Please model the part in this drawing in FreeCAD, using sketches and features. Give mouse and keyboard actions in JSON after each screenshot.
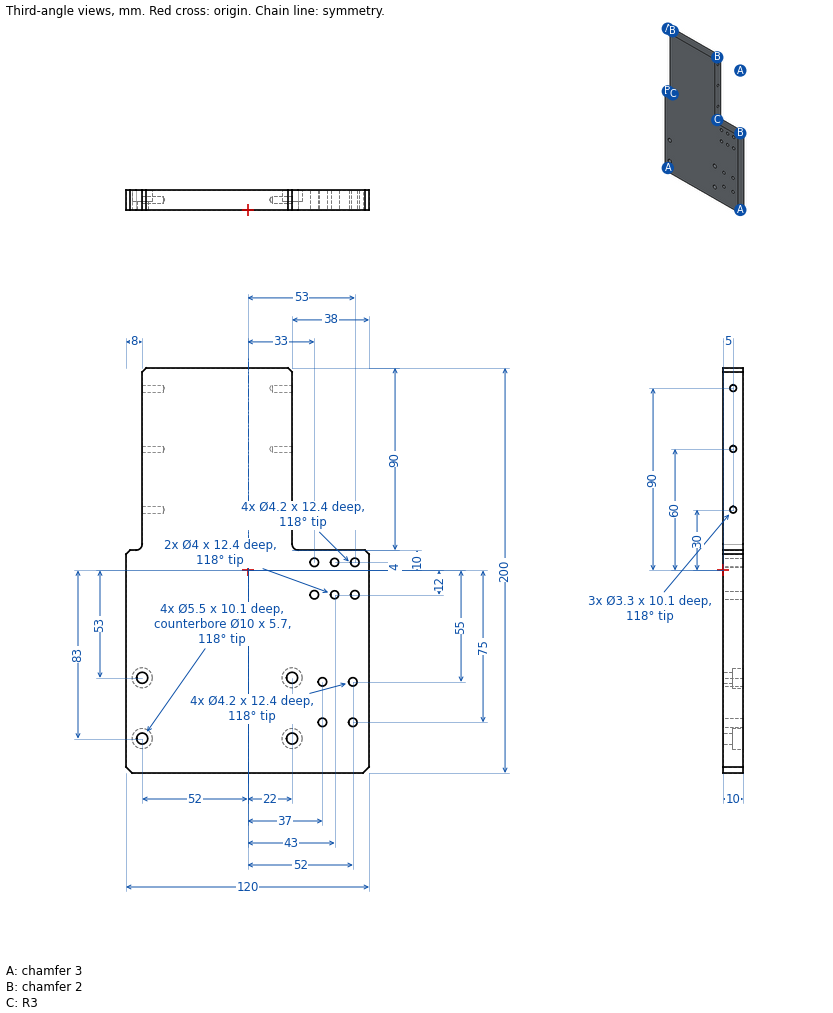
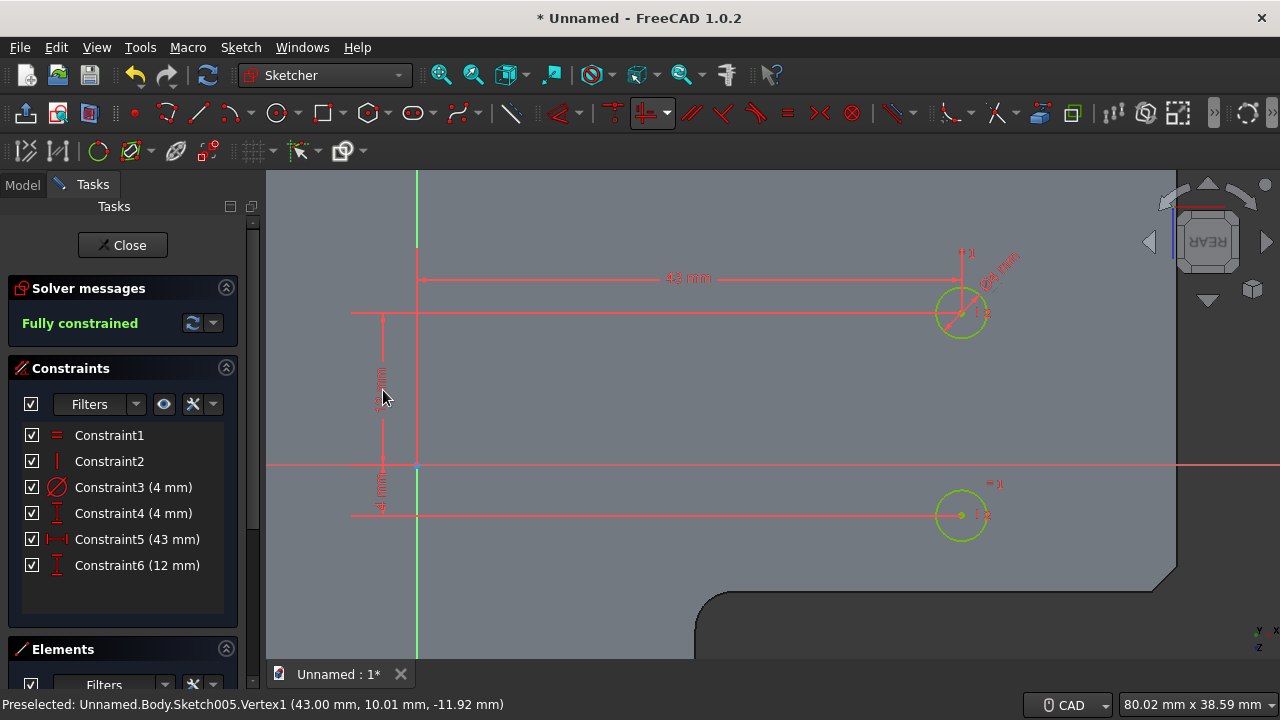
{"action": "left_click", "coordinate": [123, 245]}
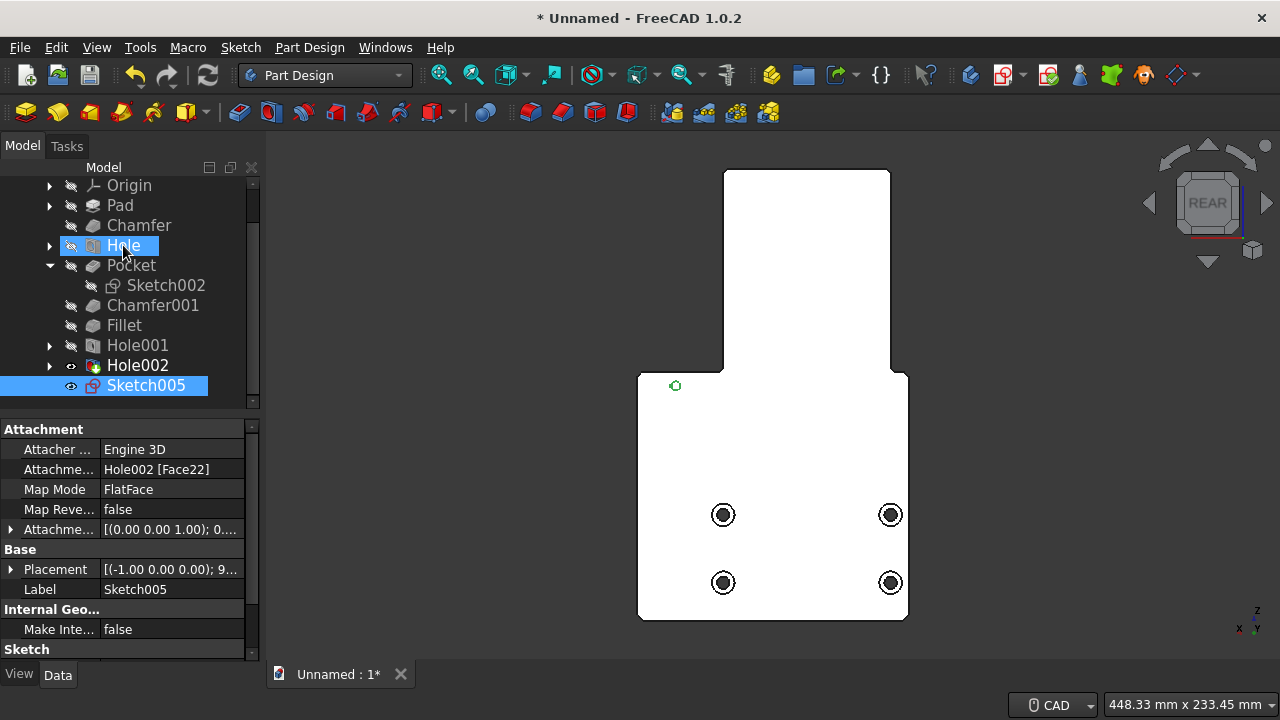
{"action": "left_click", "coordinate": [272, 112]}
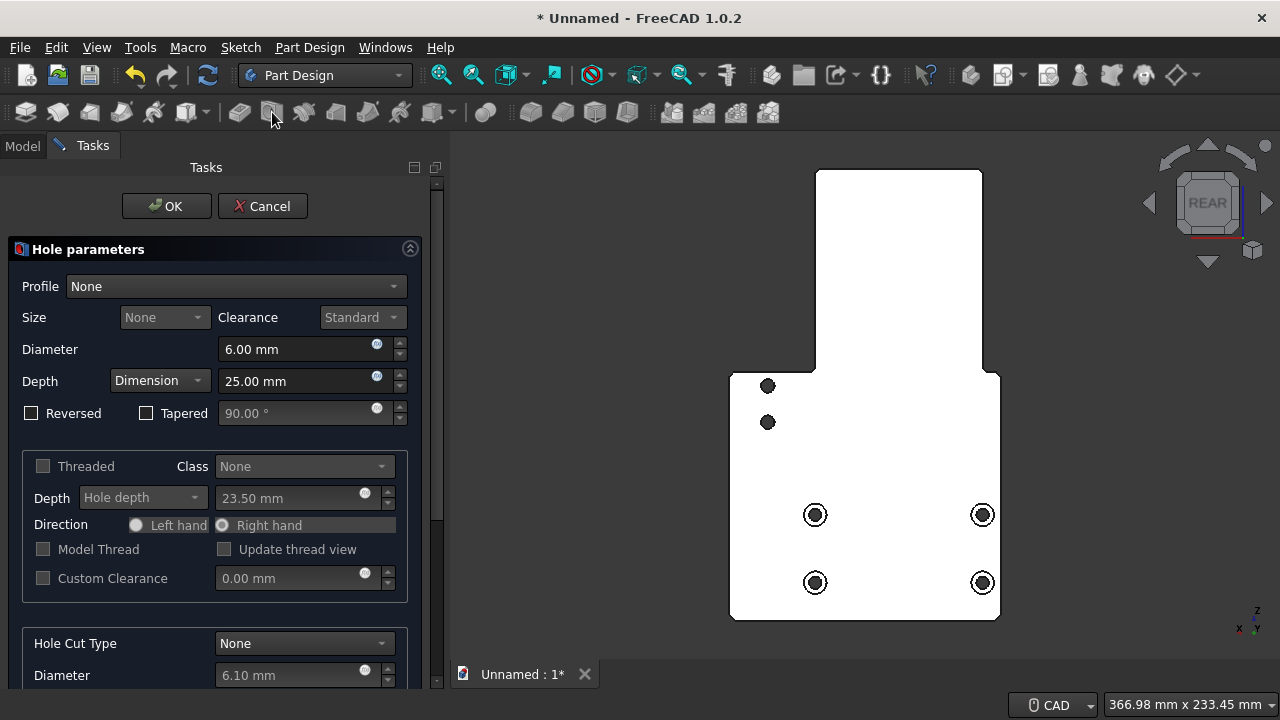
{"action": "triple_click", "coordinate": [305, 349]}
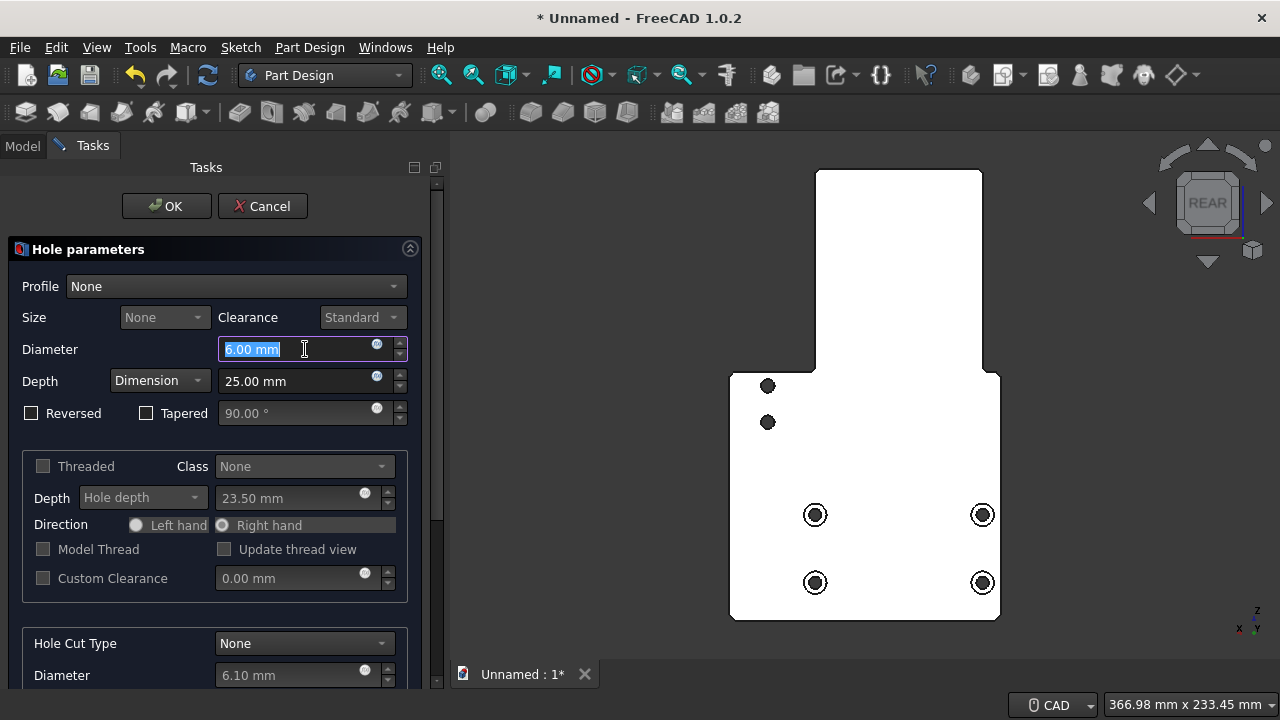
{"action": "type", "text": "4"}
{"action": "key", "text": "Tab"}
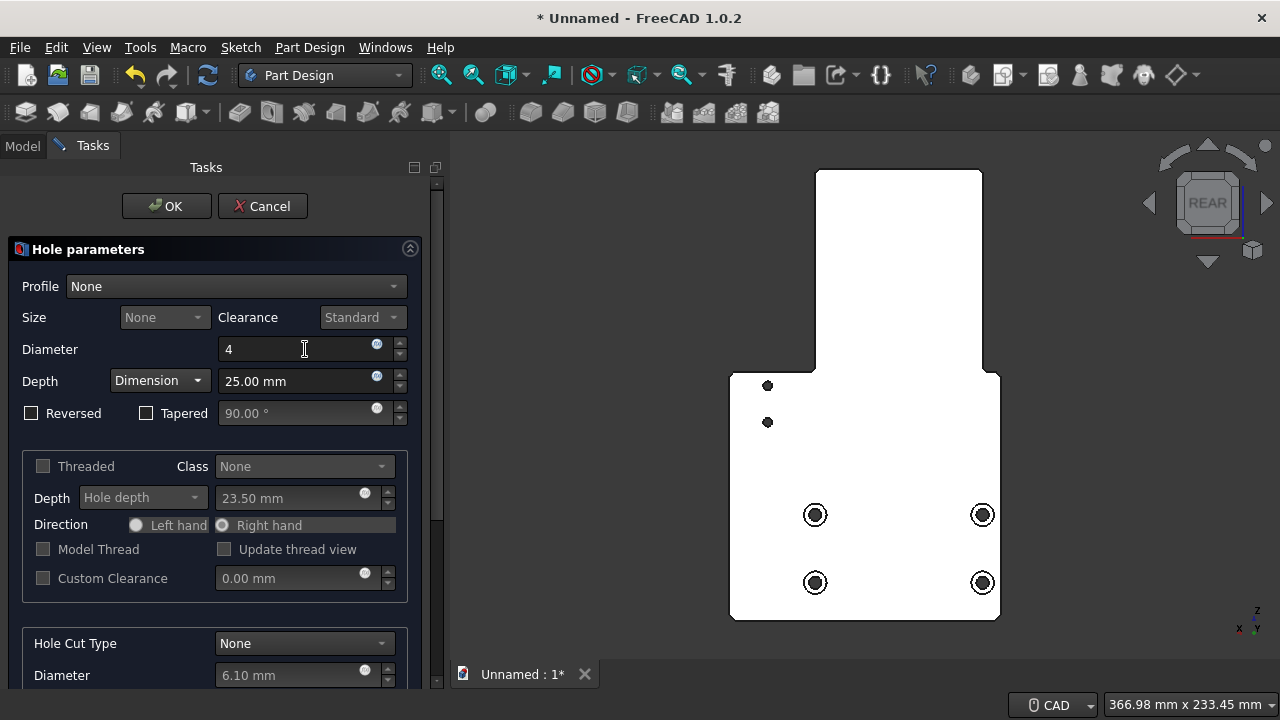
{"action": "triple_click", "coordinate": [305, 381]}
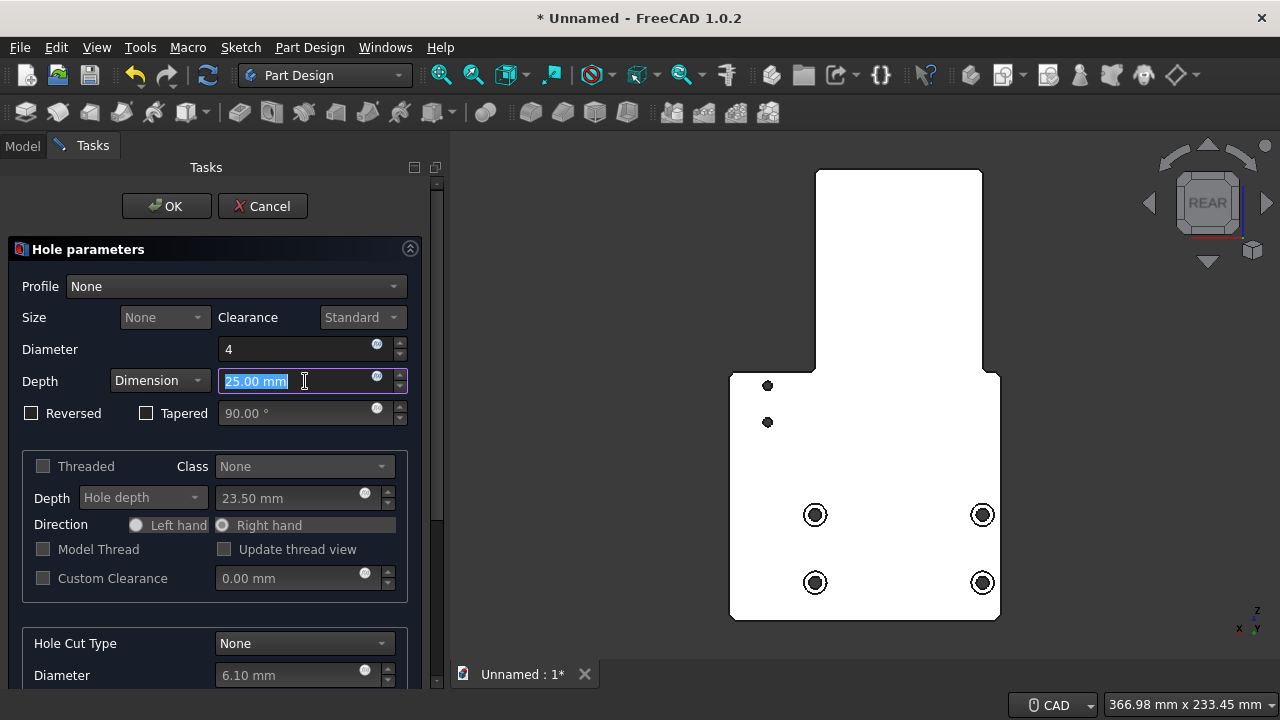
{"action": "type", "text": "12.4"}
{"action": "key", "text": "Tab"}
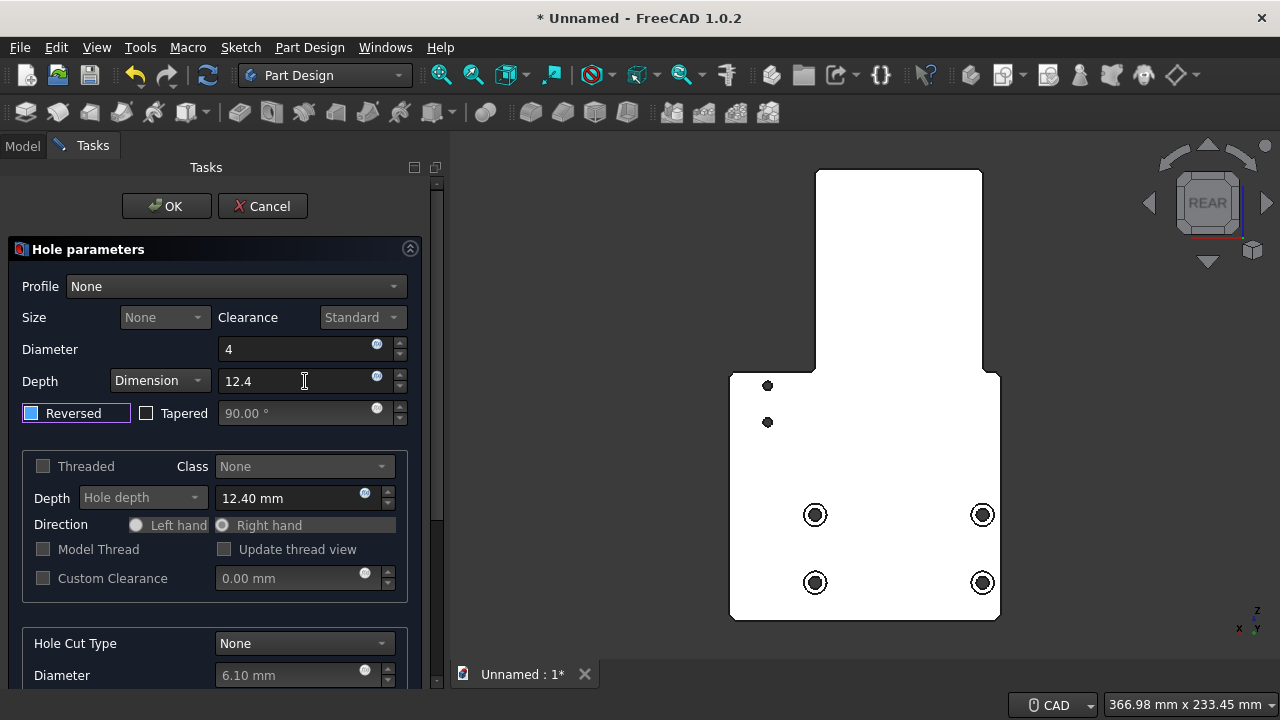
{"action": "left_click", "coordinate": [167, 206]}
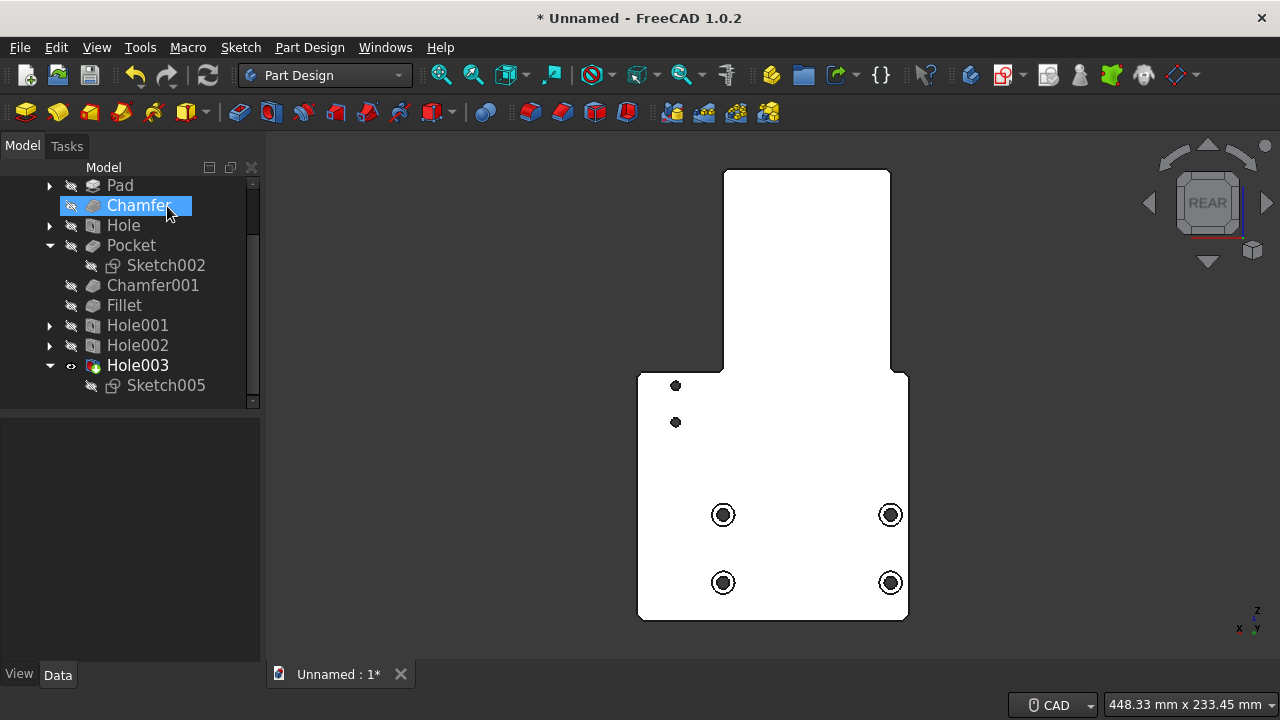
{"action": "left_click", "coordinate": [812, 459]}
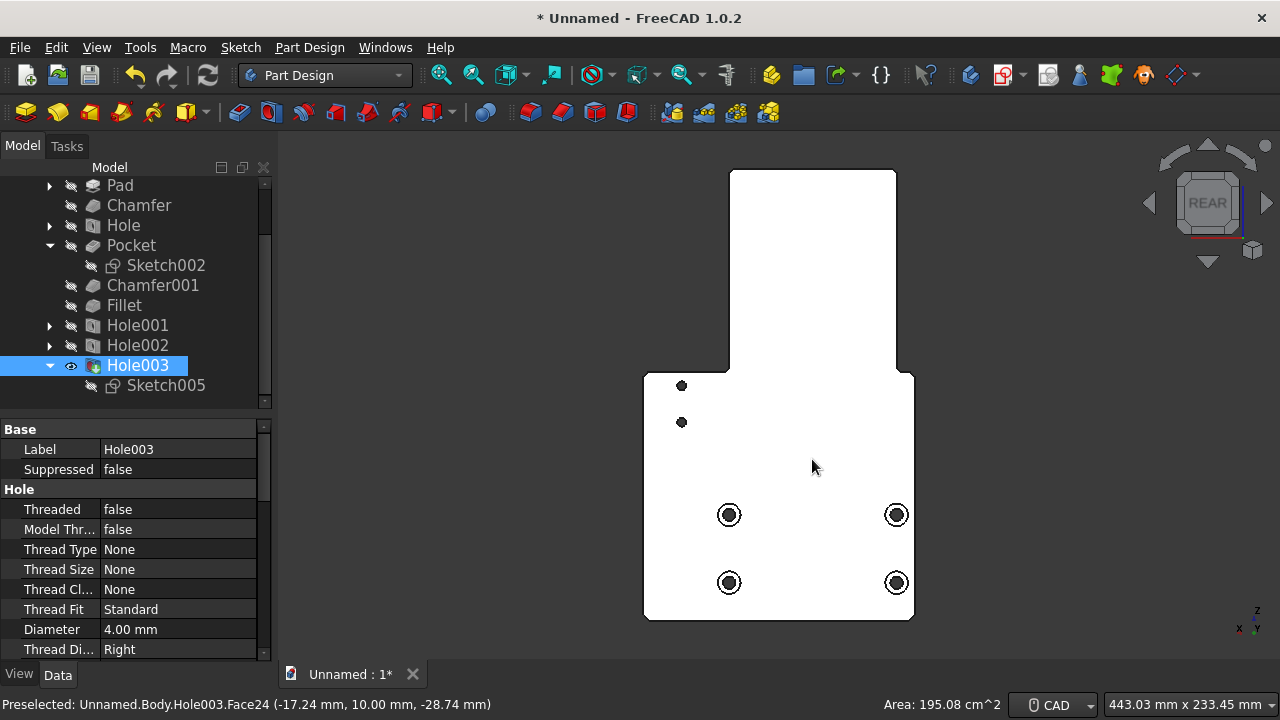
{"action": "left_click", "coordinate": [1004, 76]}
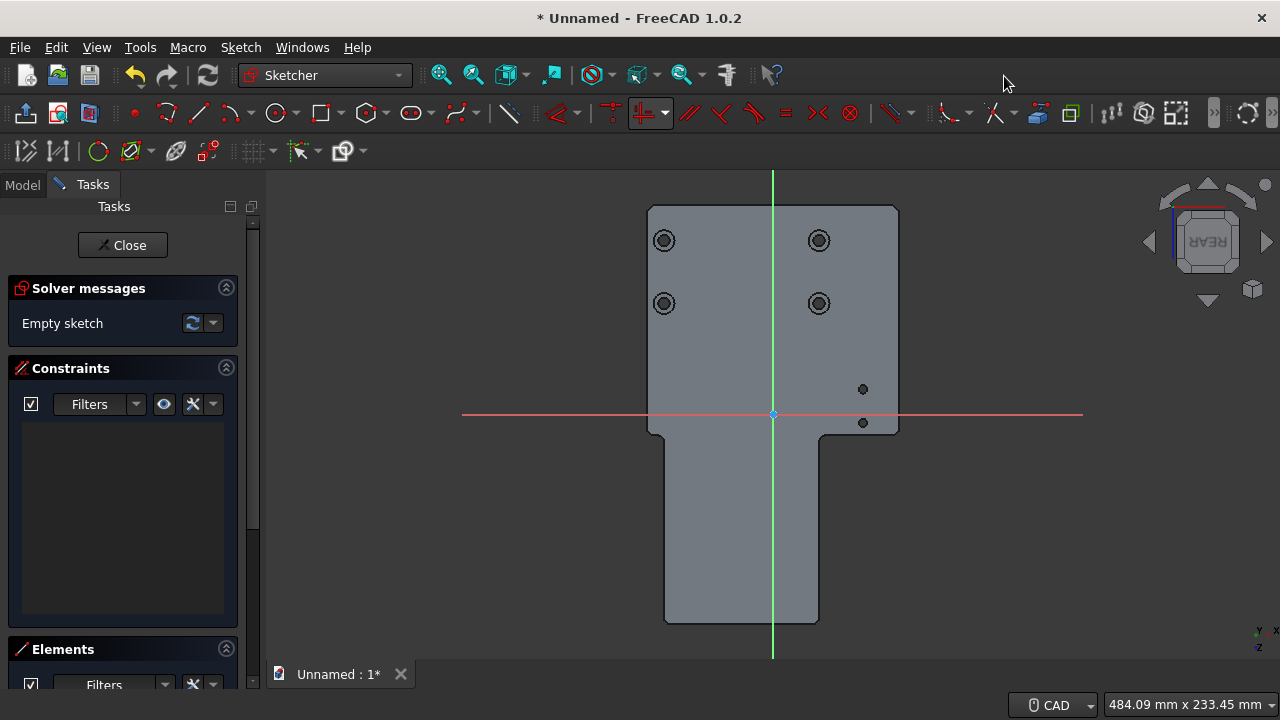
{"action": "scroll", "coordinate": [863, 404], "scroll_direction": "up", "scroll_amount": 8}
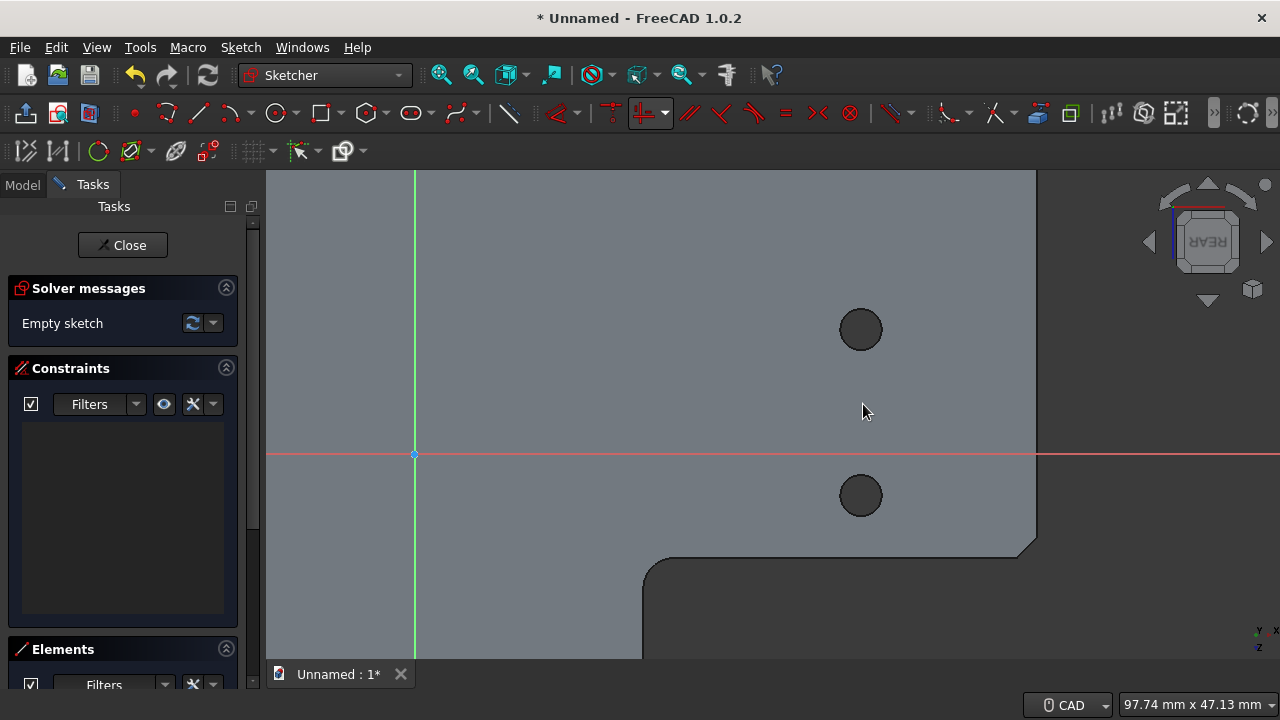
{"action": "left_click", "coordinate": [276, 114]}